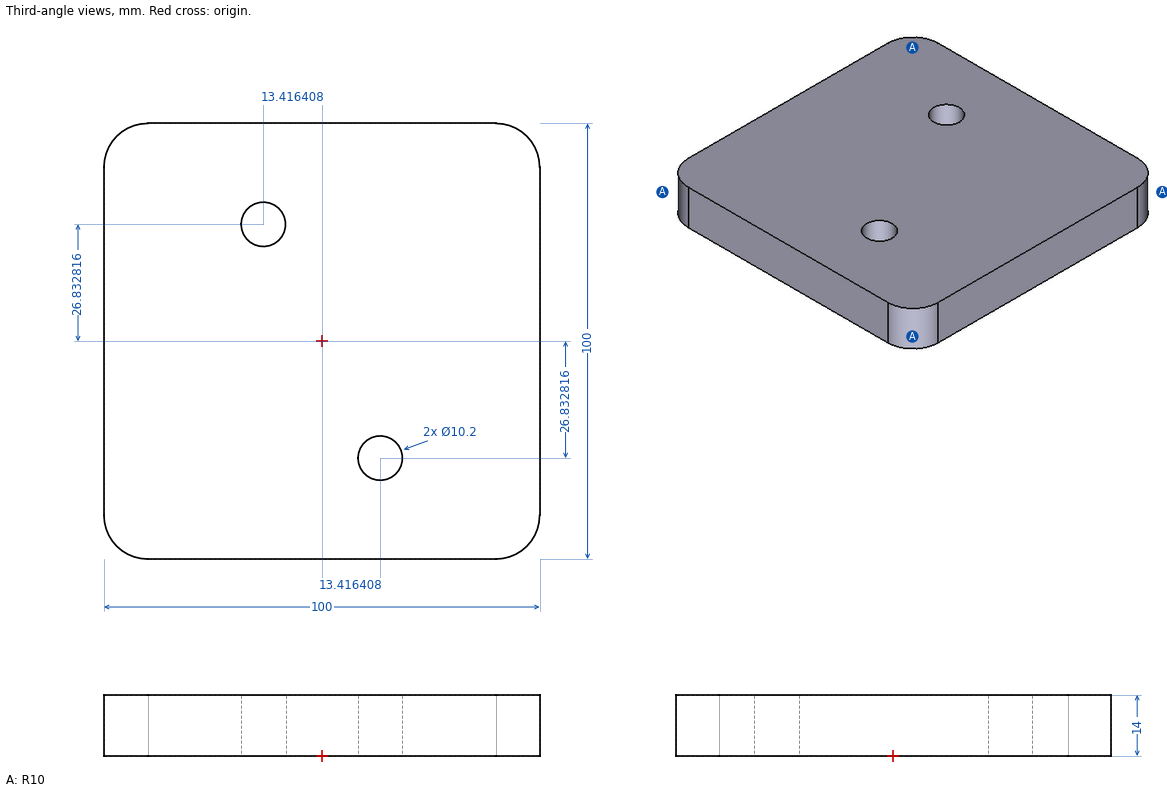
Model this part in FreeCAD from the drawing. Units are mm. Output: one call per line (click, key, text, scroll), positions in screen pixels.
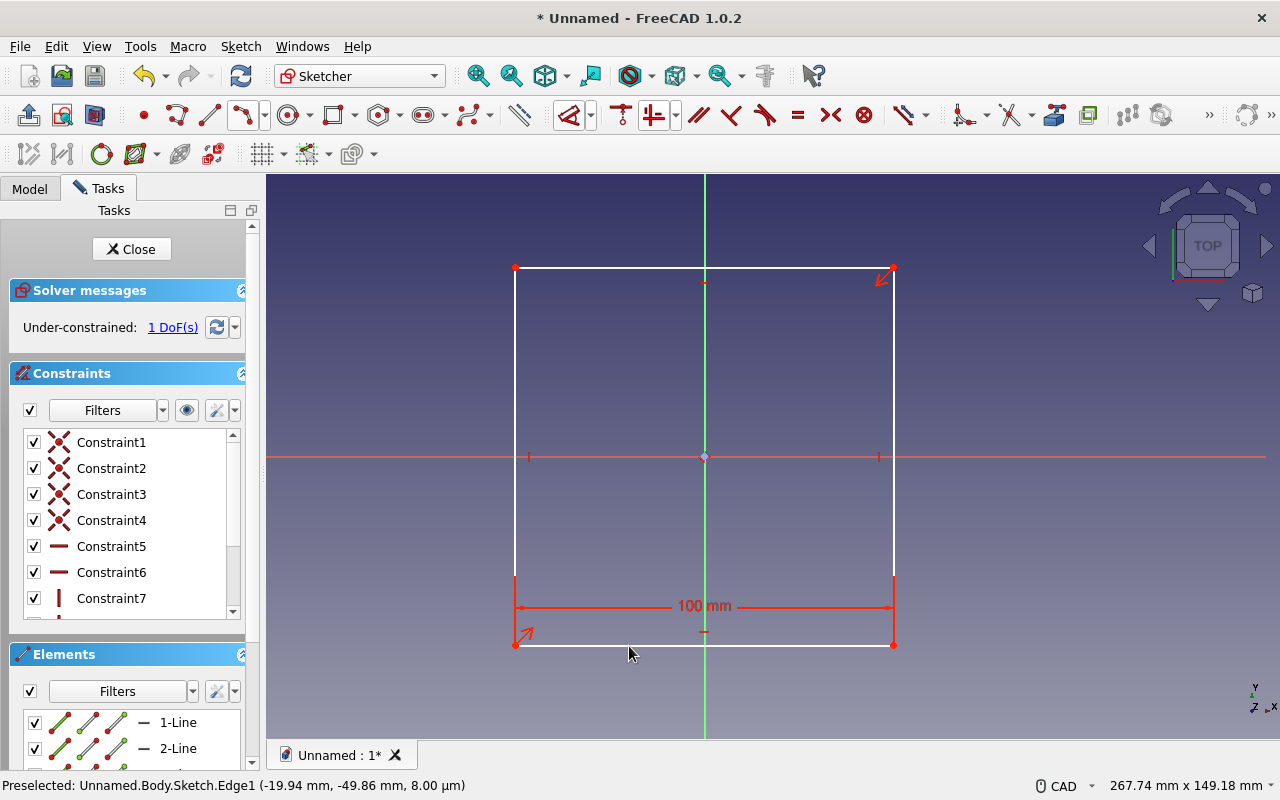
click(894, 532)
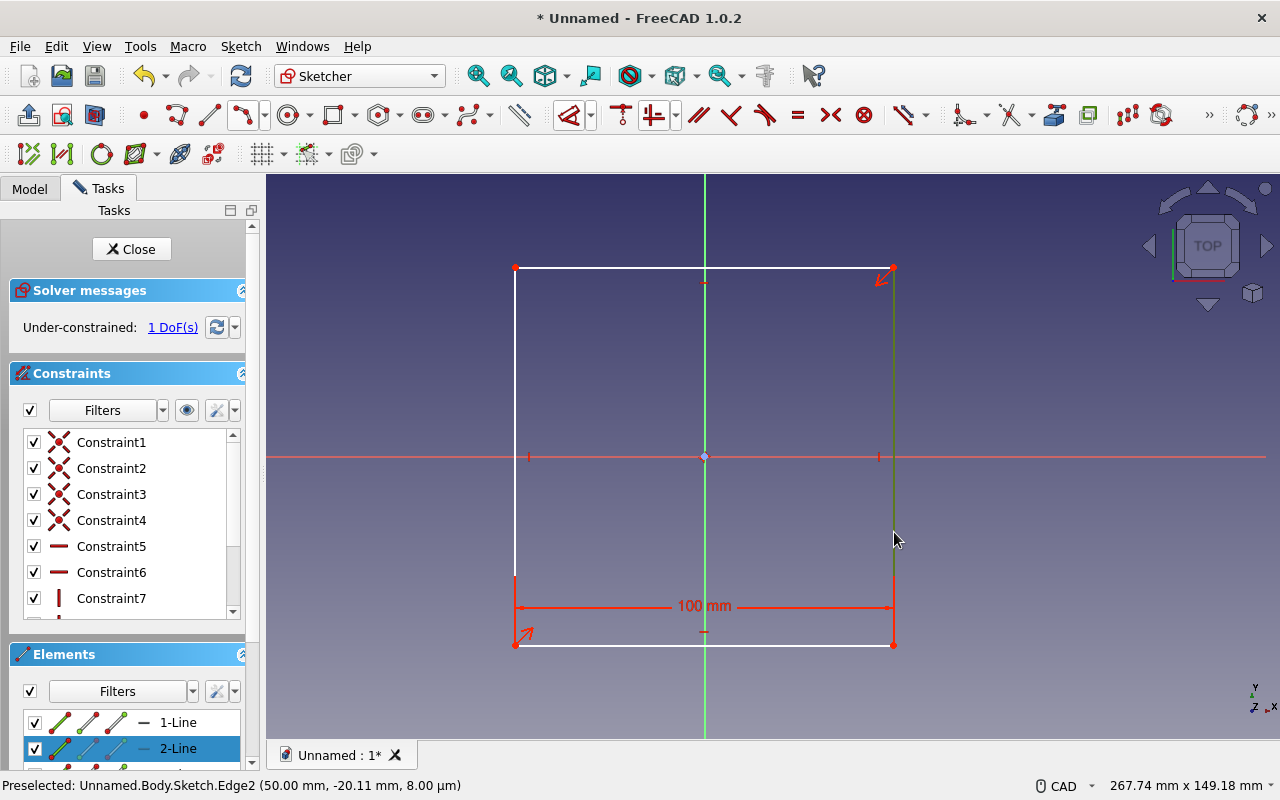
click(590, 116)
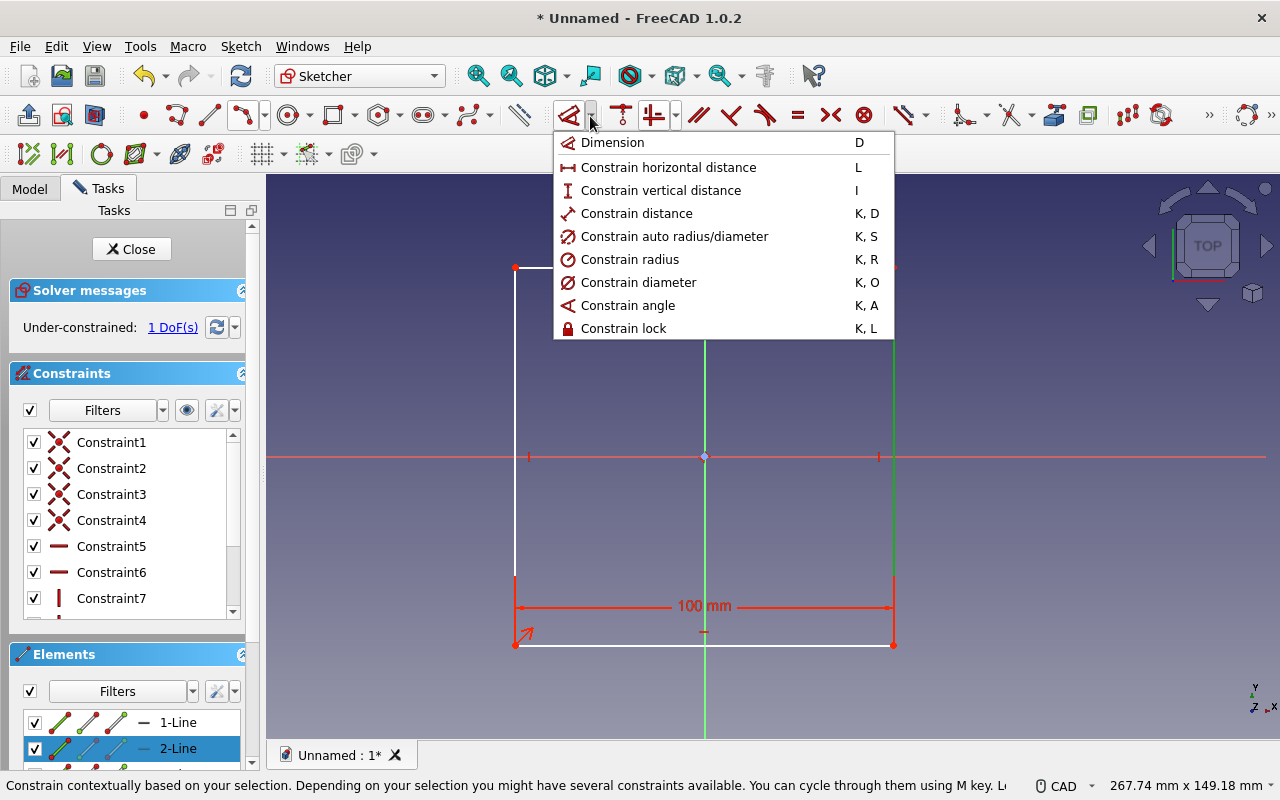
click(724, 190)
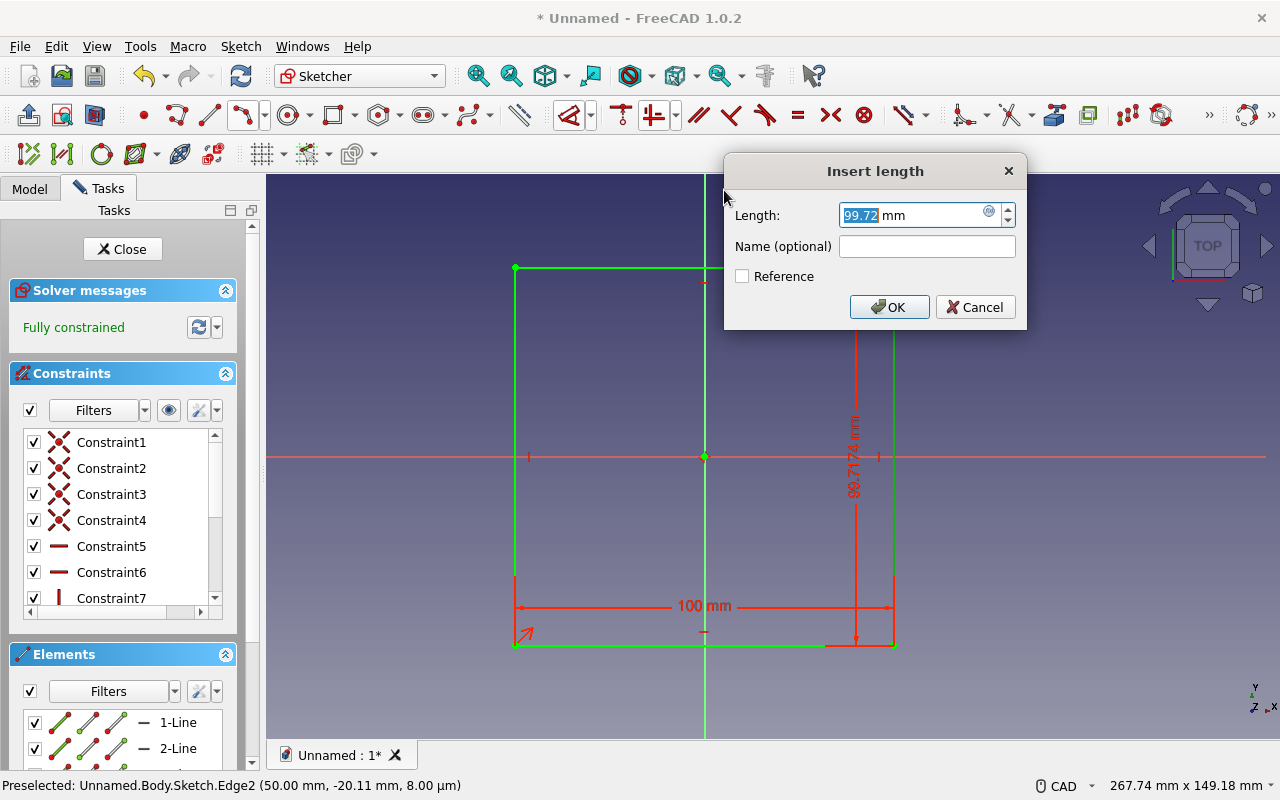
text(100)
key(Return)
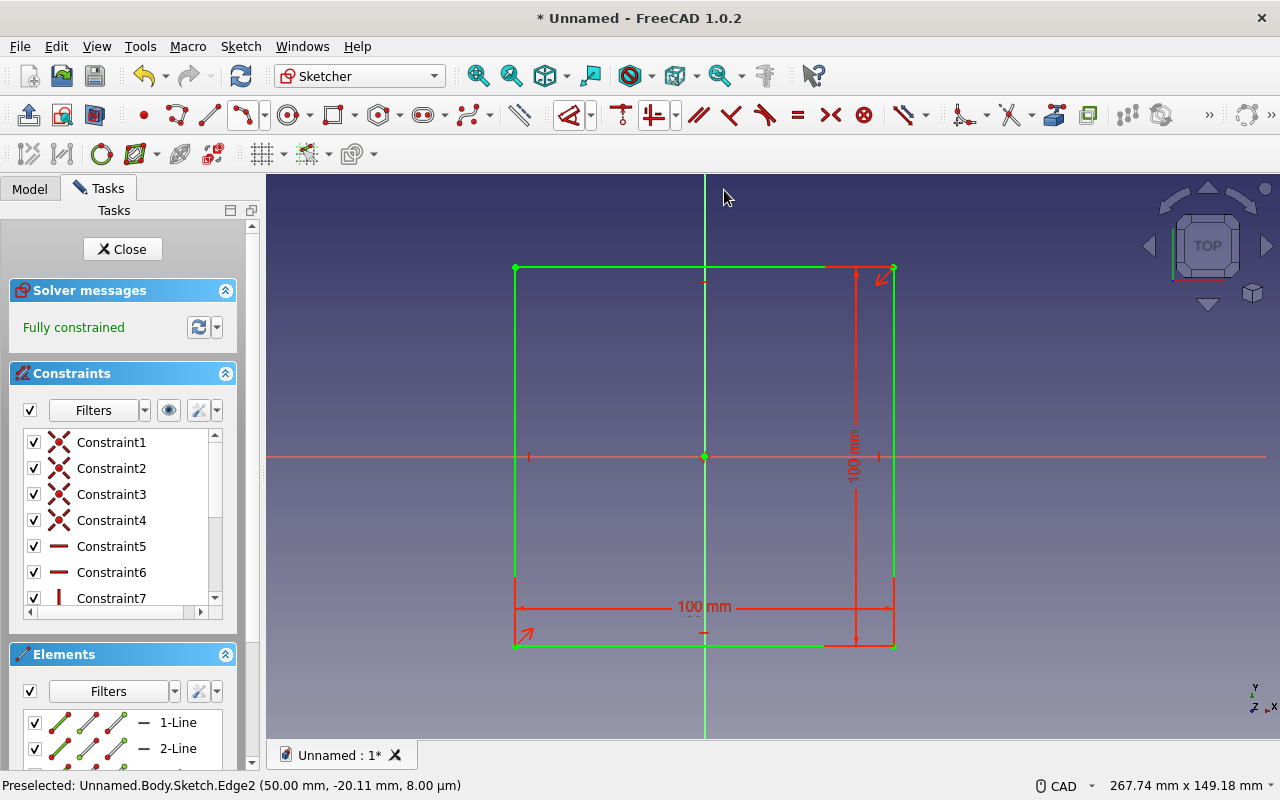
click(123, 249)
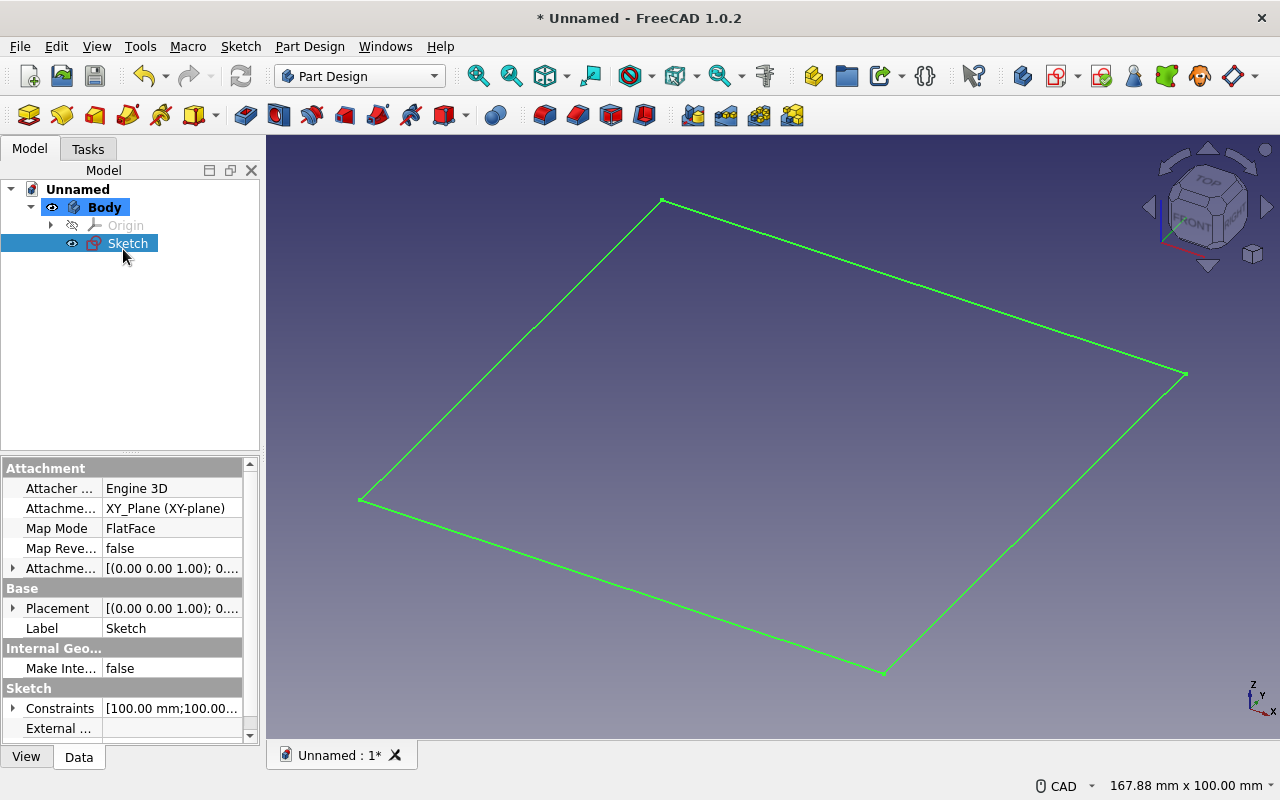
click(29, 116)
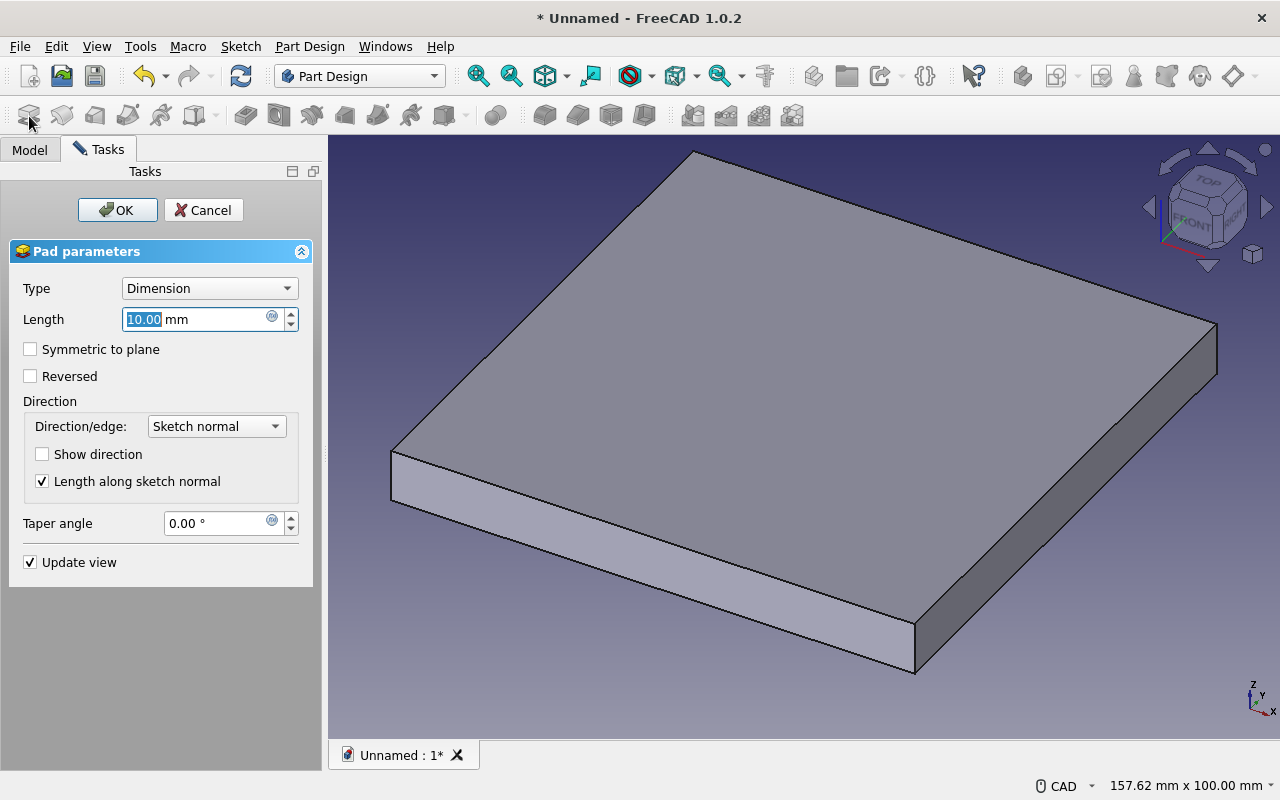
text(14)
key(Tab)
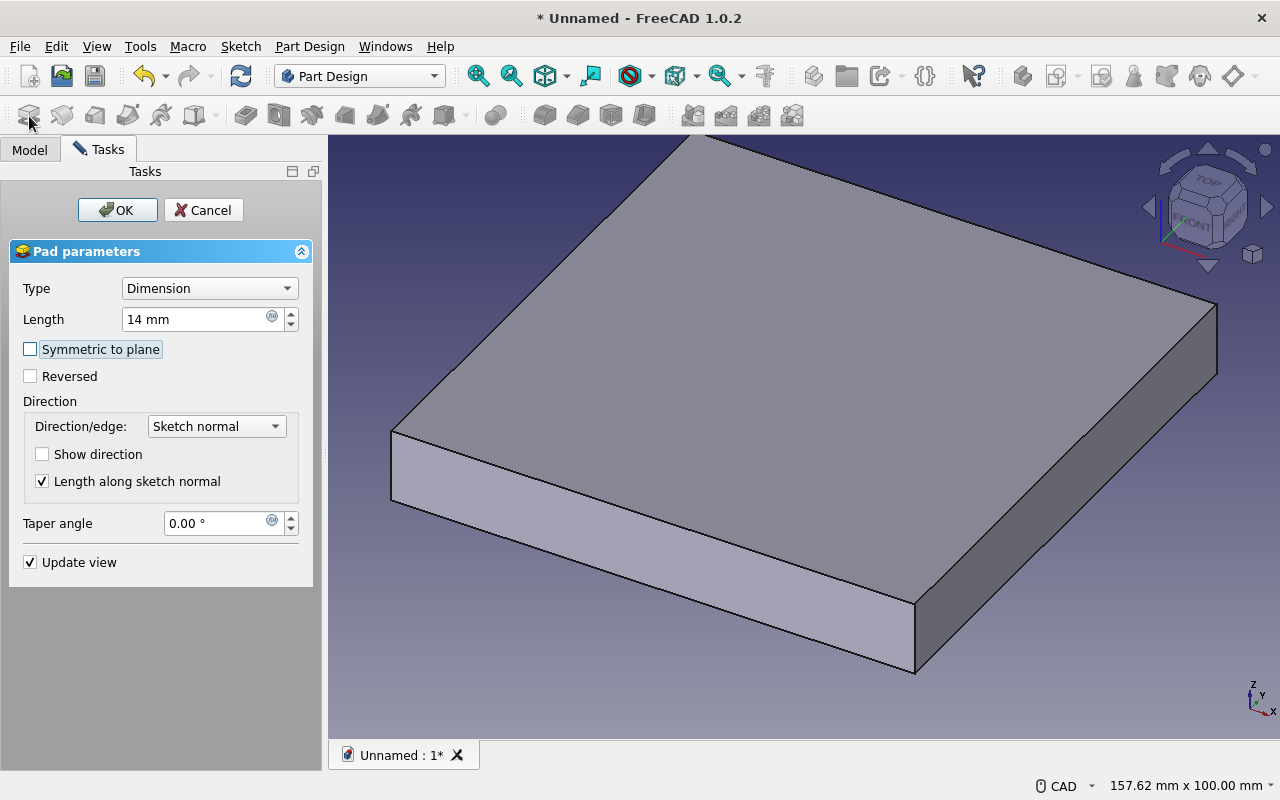
click(118, 210)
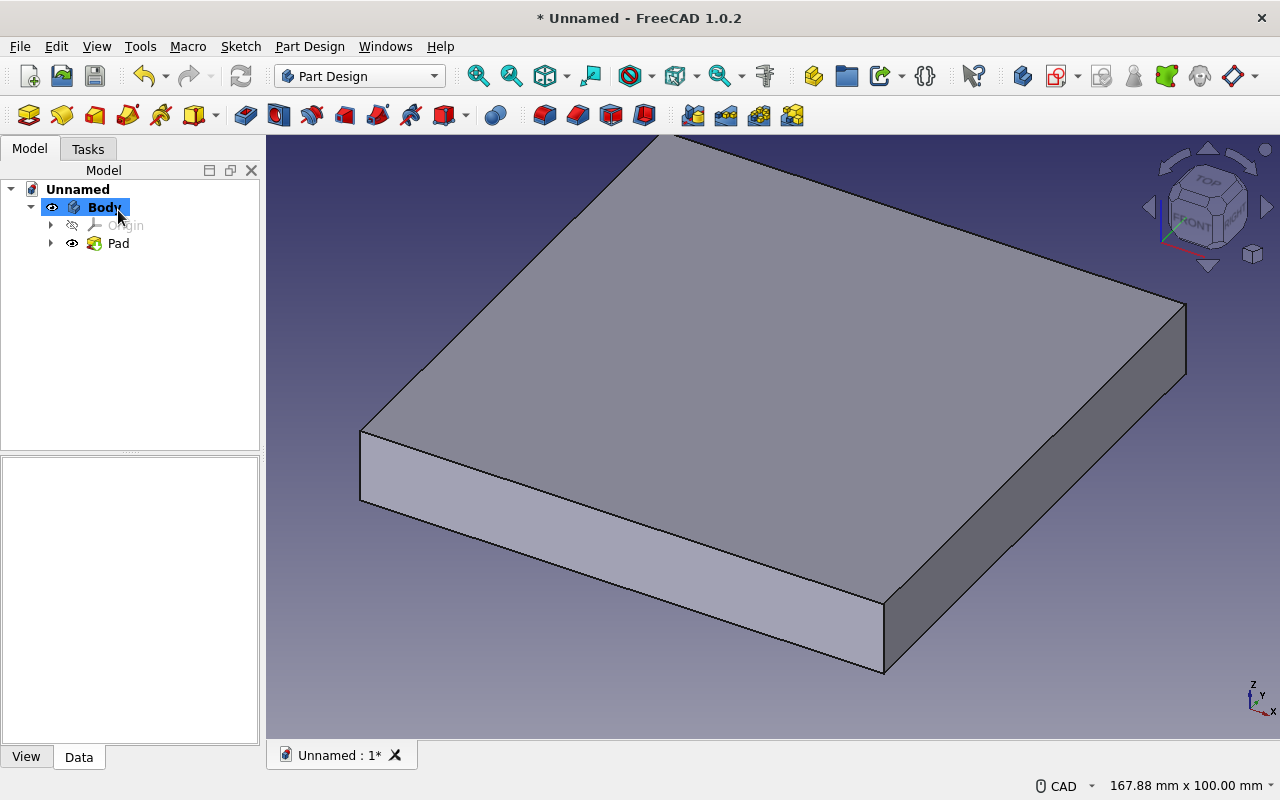
click(479, 76)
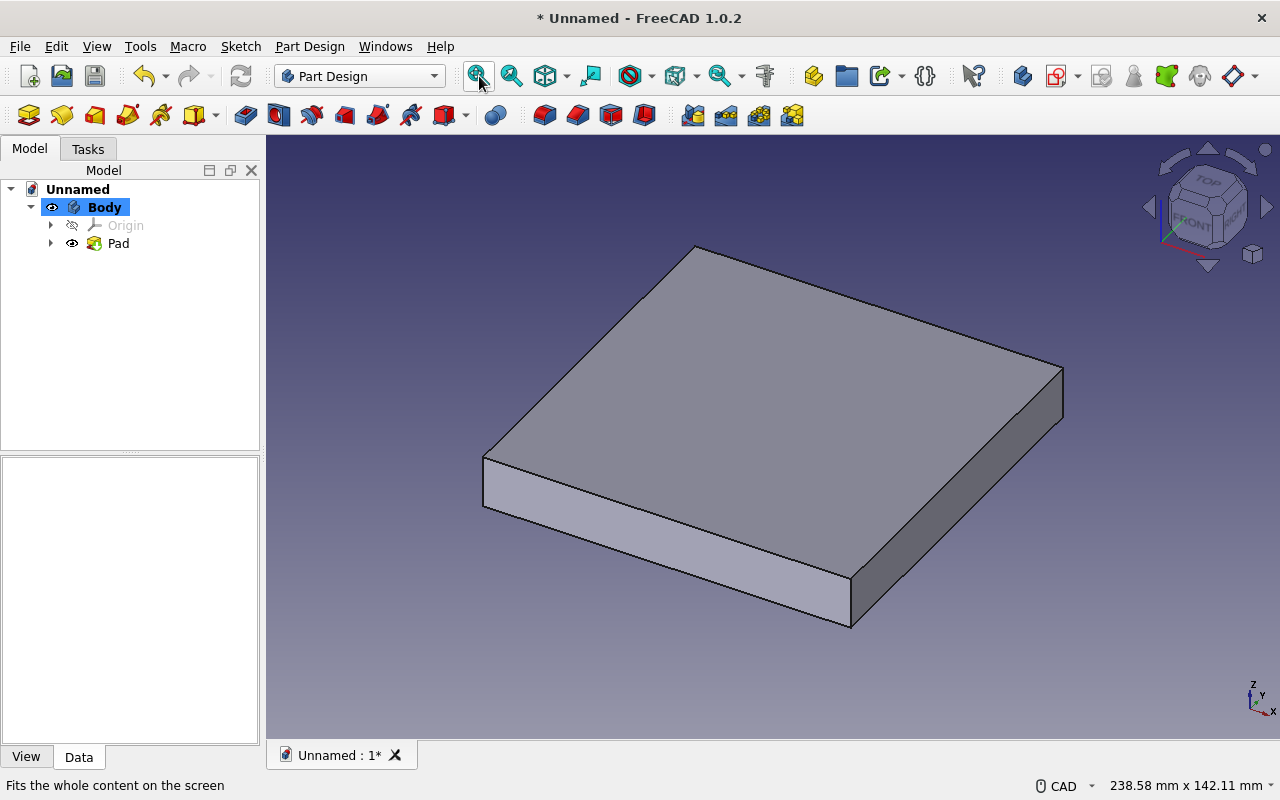
click(773, 412)